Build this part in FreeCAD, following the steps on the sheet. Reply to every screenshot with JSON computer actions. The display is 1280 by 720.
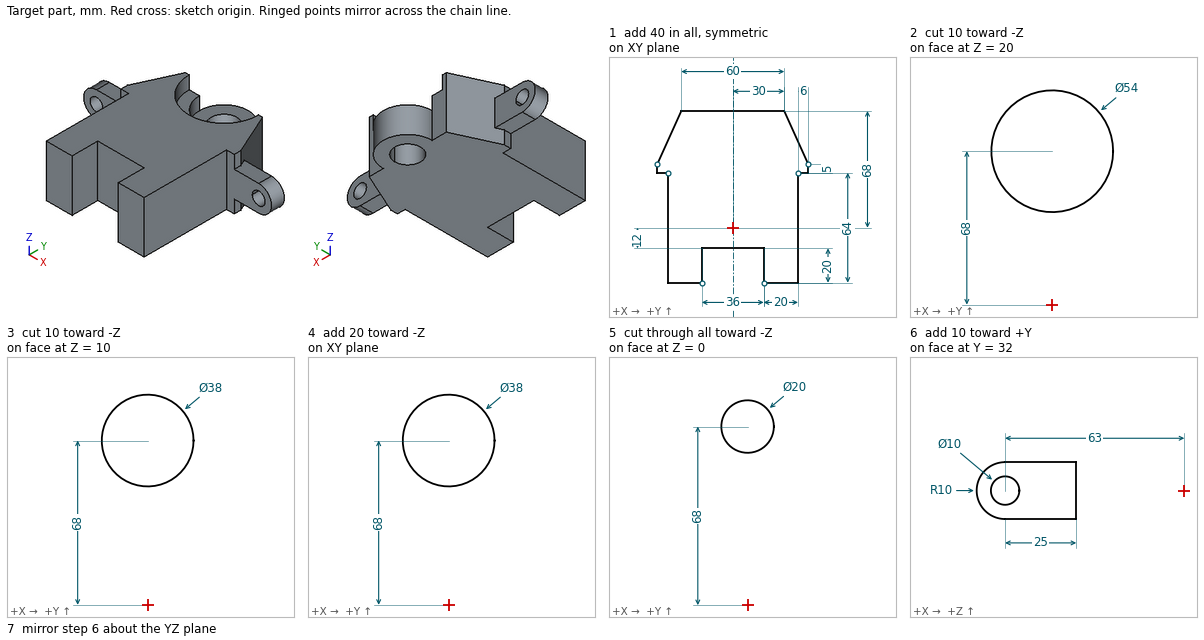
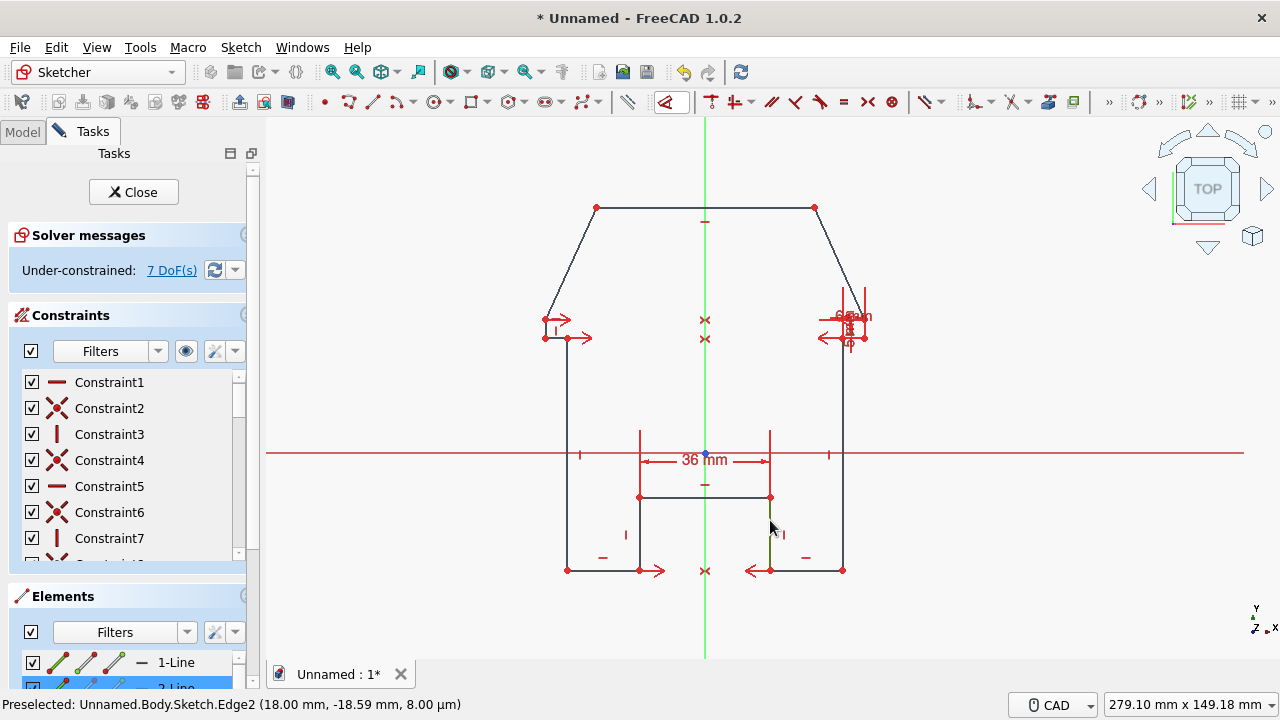
{"action": "left_click", "coordinate": [684, 102]}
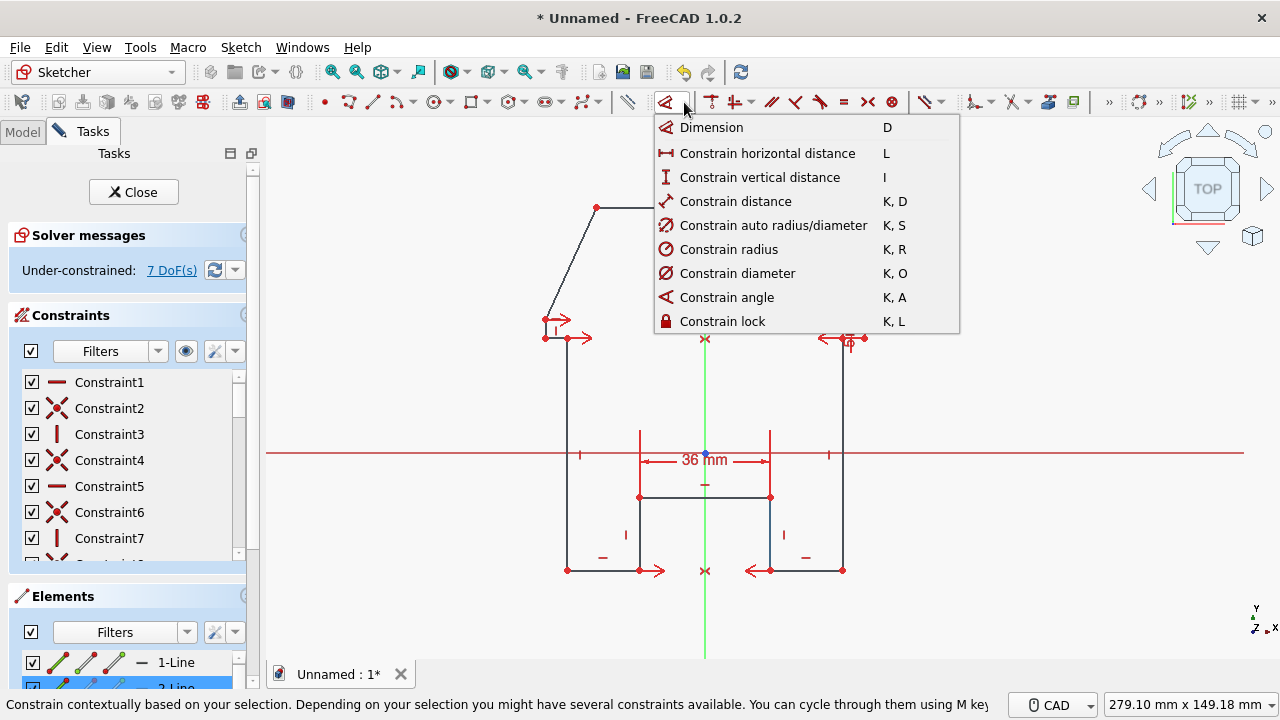
{"action": "left_click", "coordinate": [807, 177]}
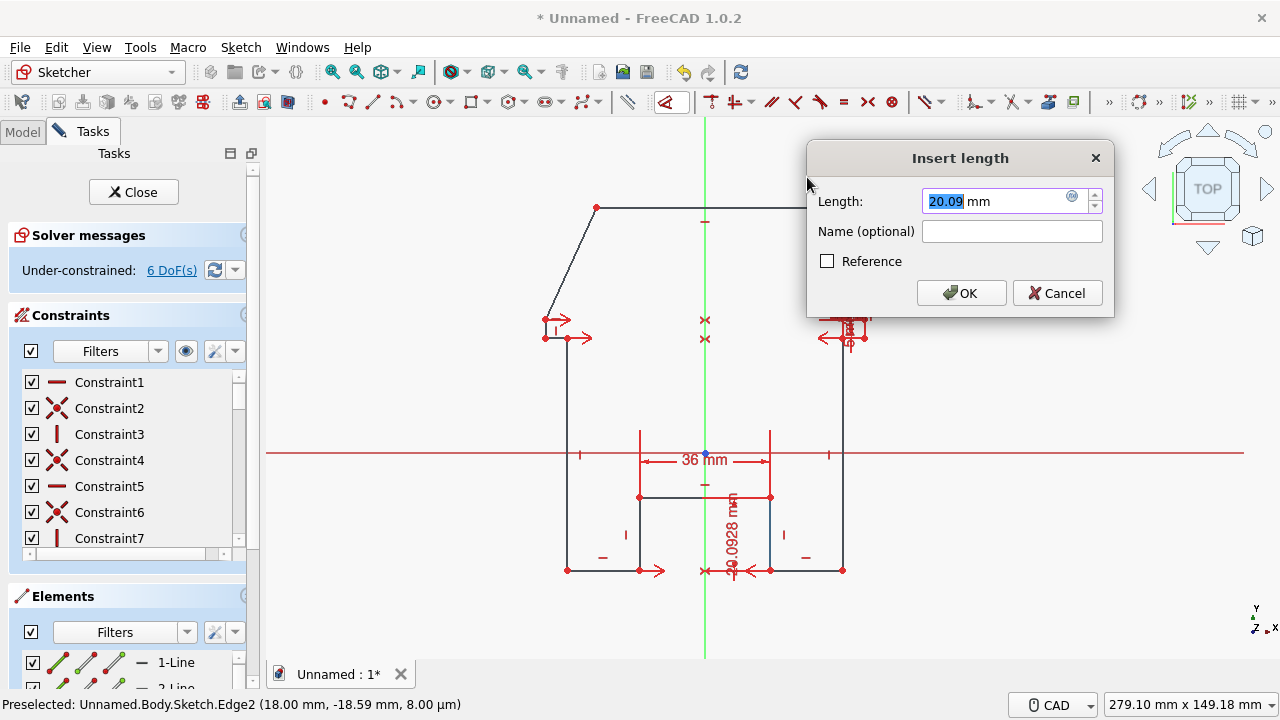
{"action": "type", "text": "20"}
{"action": "key", "text": "Return"}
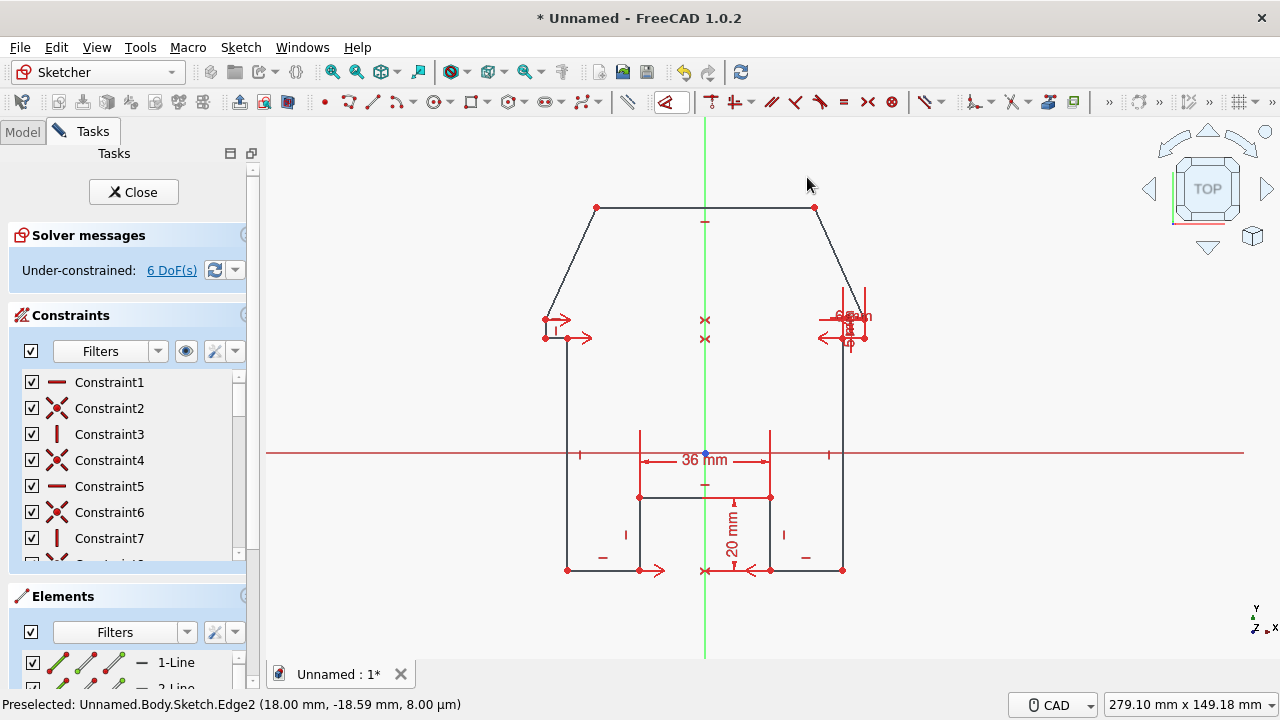
{"action": "left_click", "coordinate": [792, 571]}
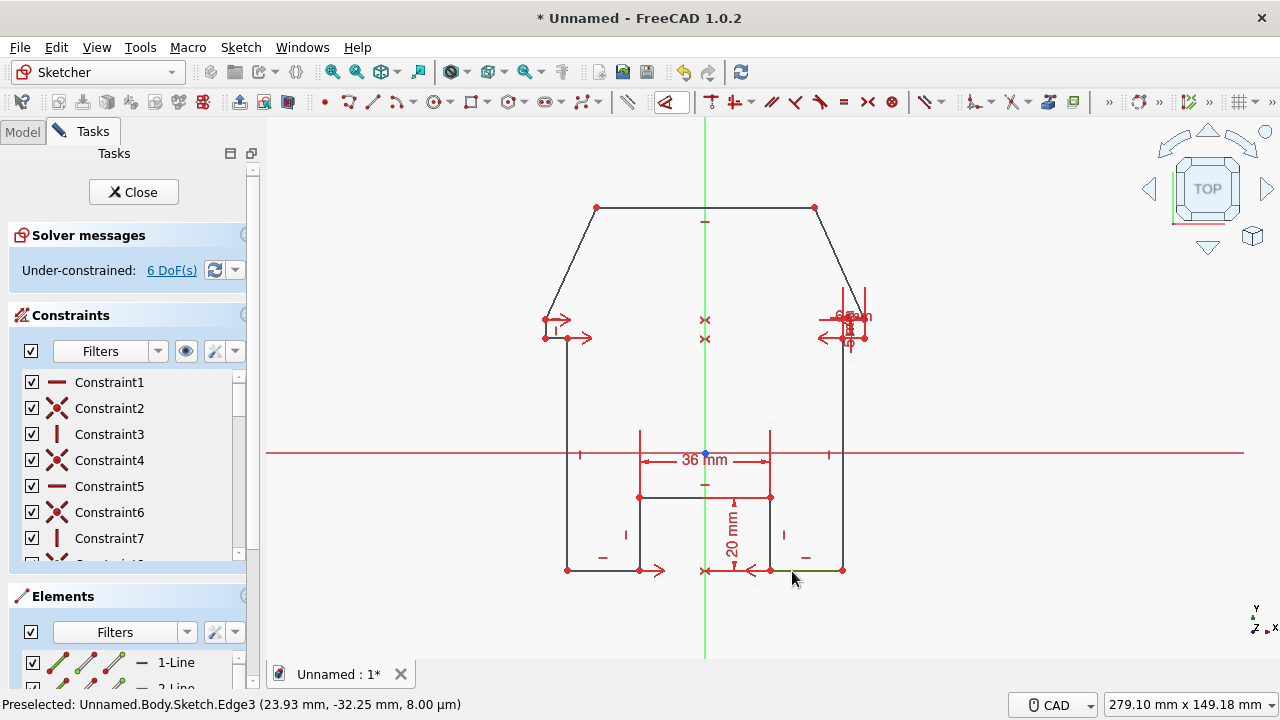
{"action": "key", "text": "l"}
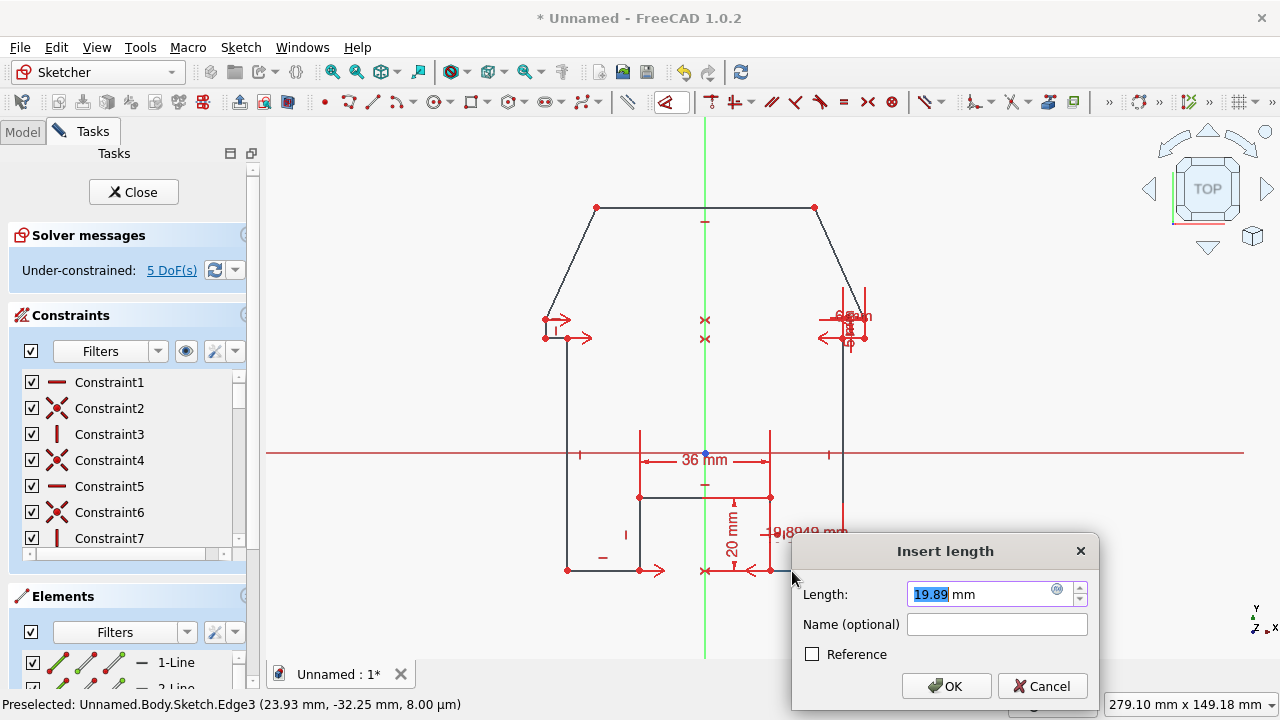
{"action": "type", "text": "20"}
{"action": "key", "text": "Return"}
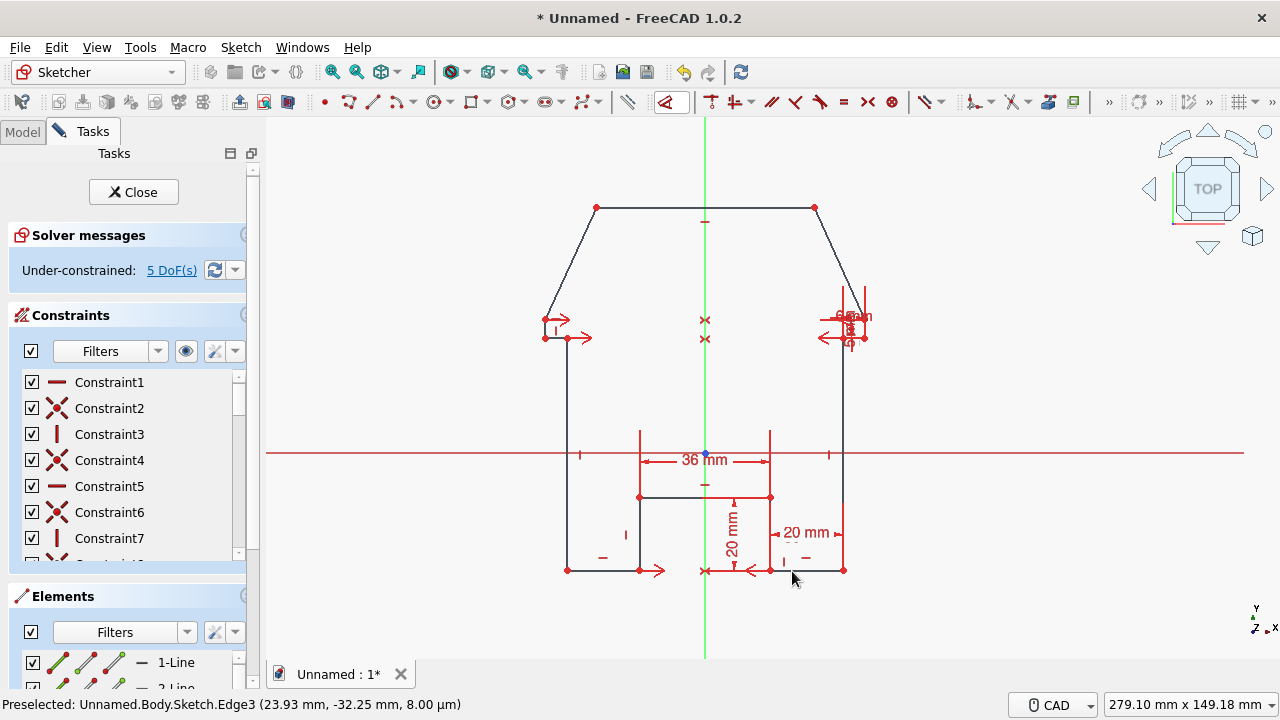
{"action": "left_click", "coordinate": [843, 501]}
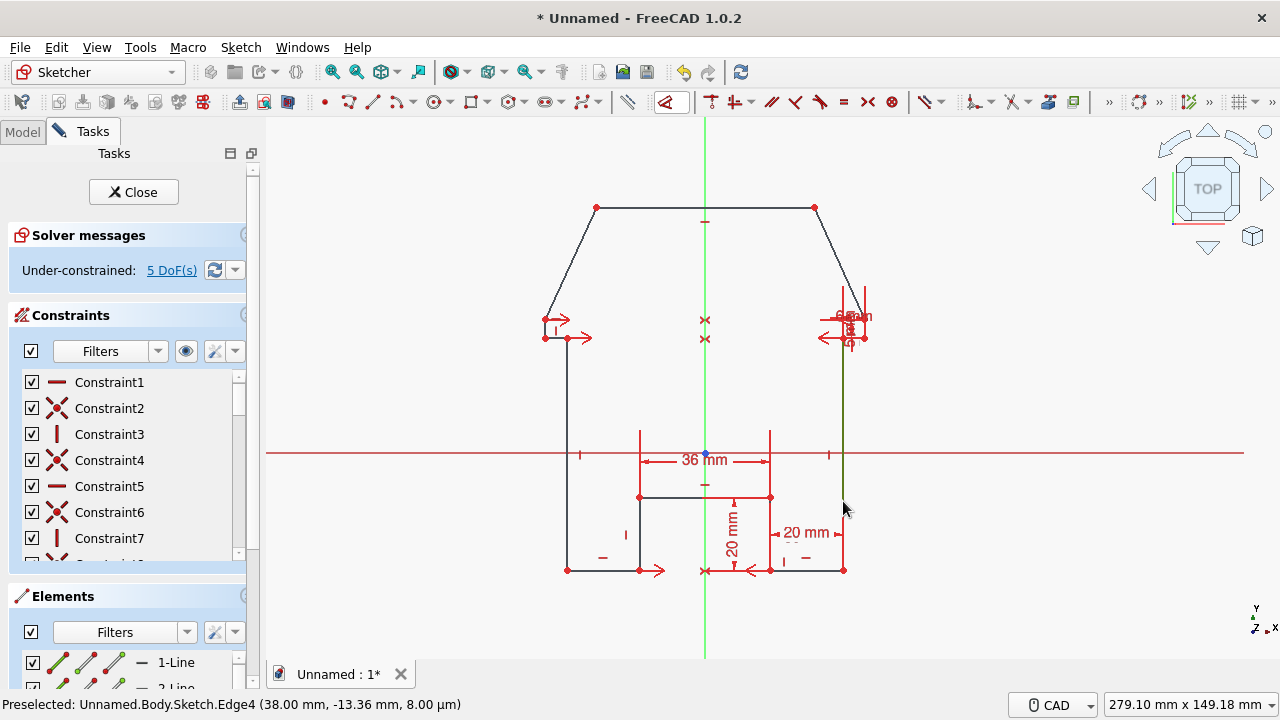
{"action": "left_click", "coordinate": [684, 102]}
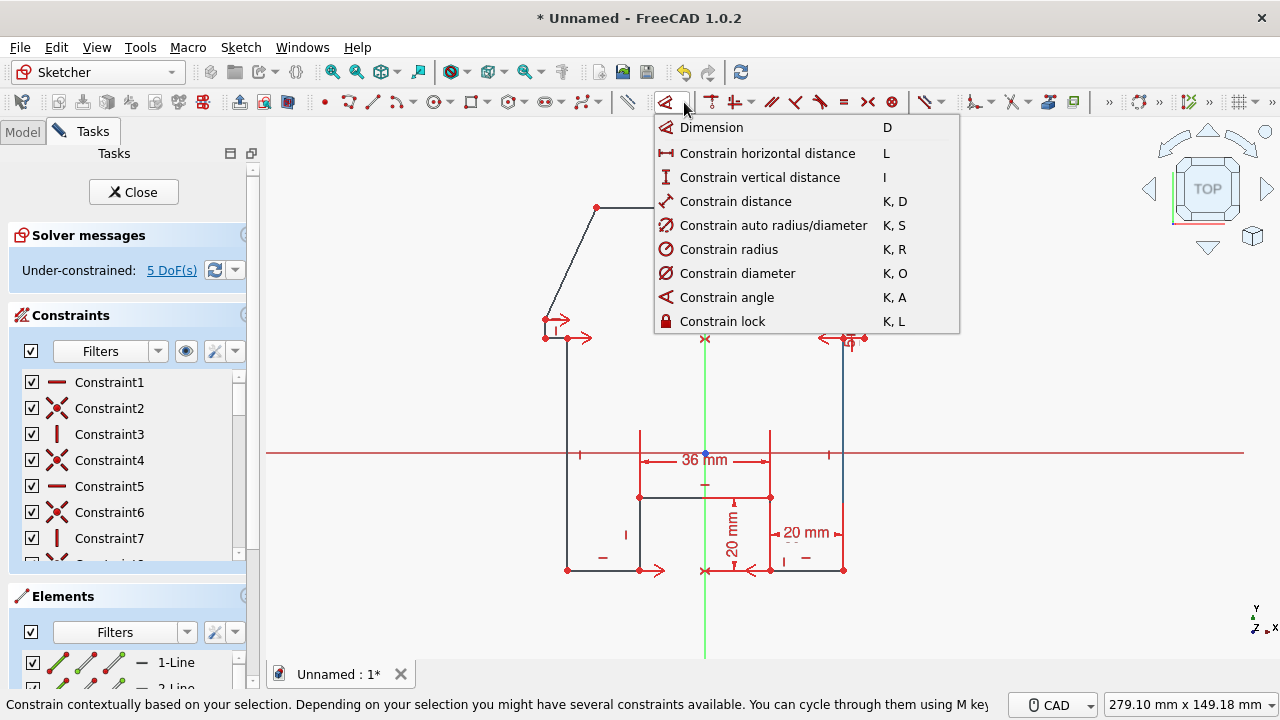
{"action": "left_click", "coordinate": [807, 177]}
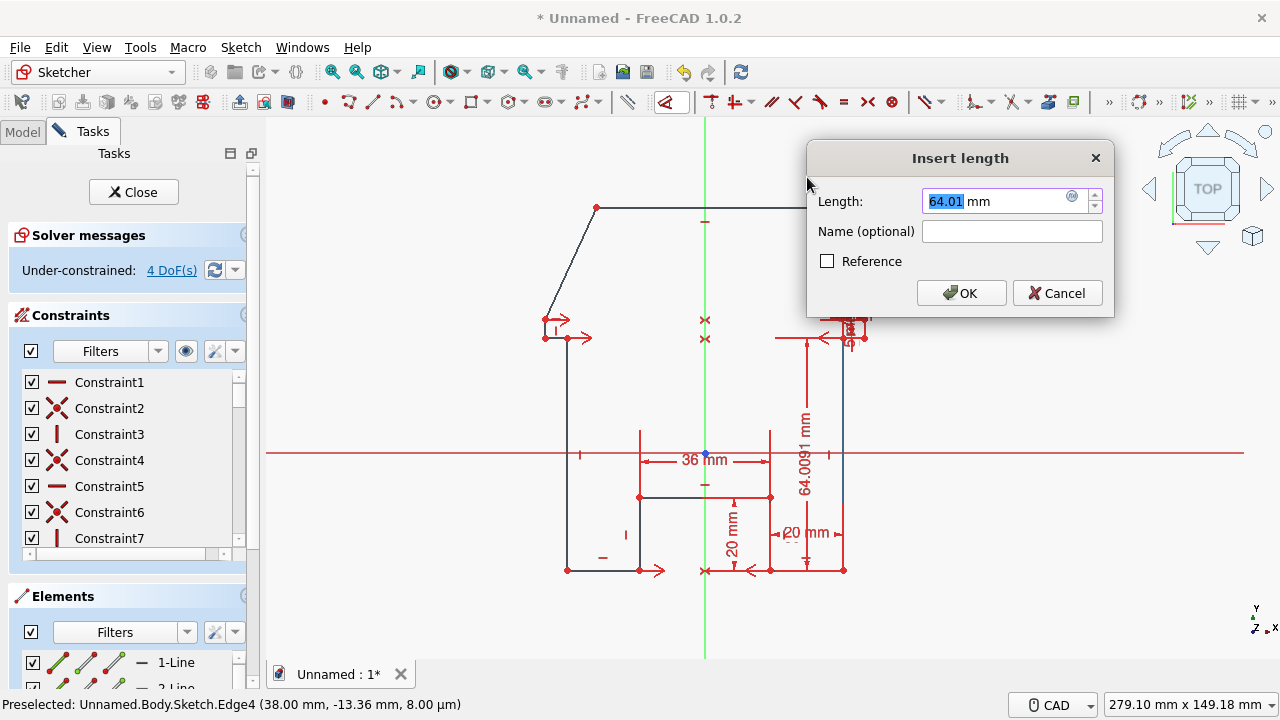
{"action": "type", "text": "64"}
{"action": "key", "text": "Return"}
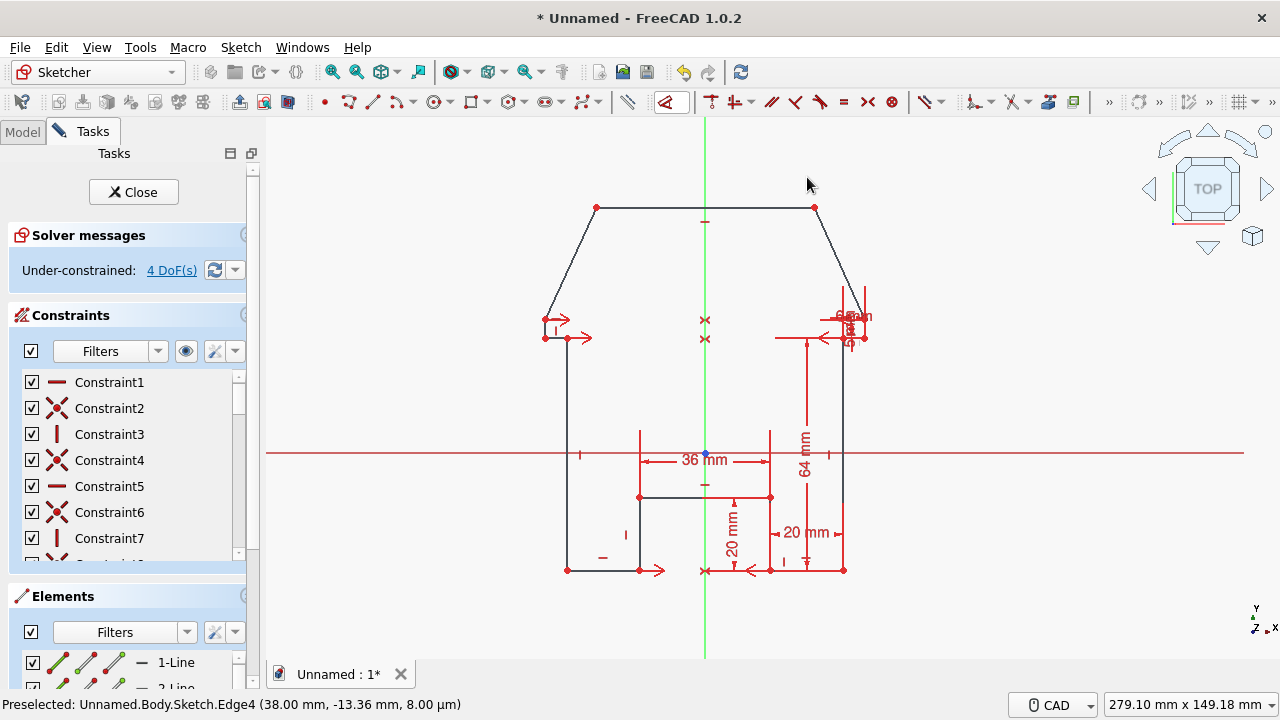
{"action": "left_click", "coordinate": [749, 208]}